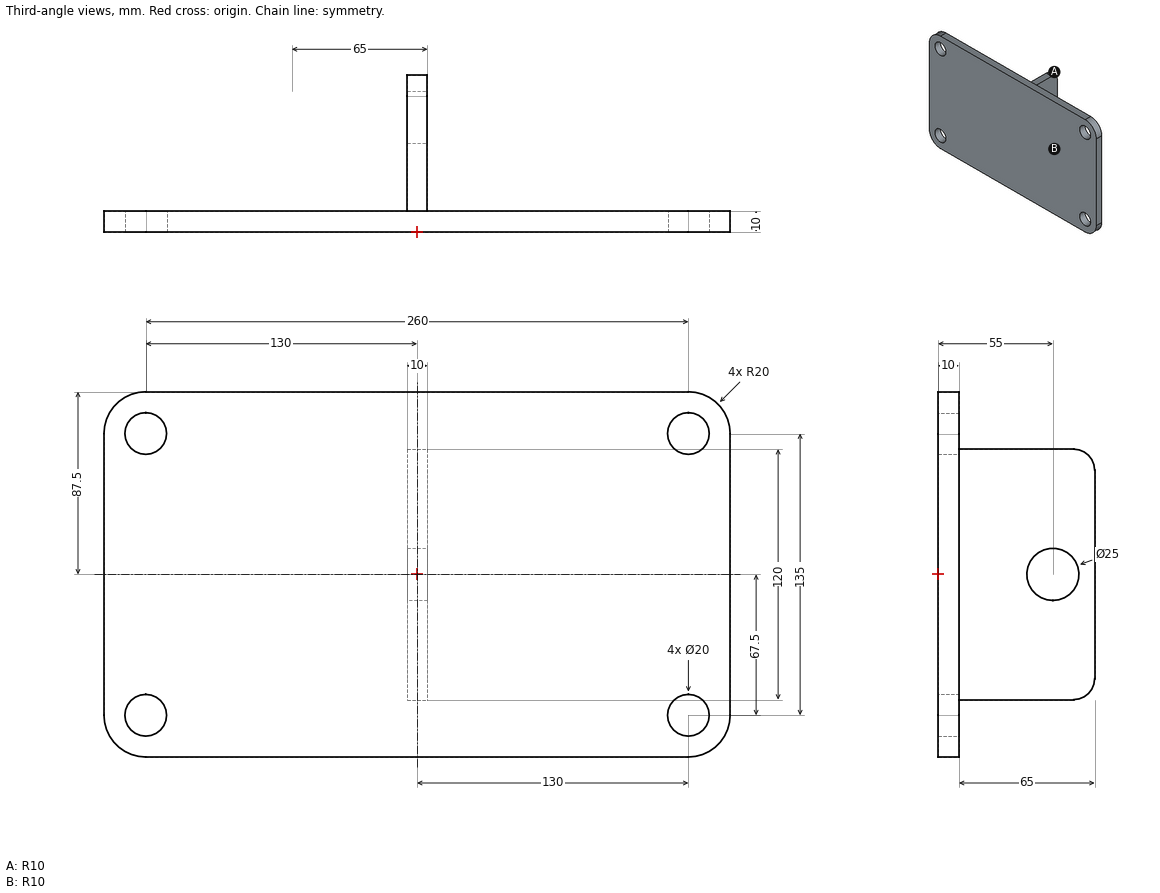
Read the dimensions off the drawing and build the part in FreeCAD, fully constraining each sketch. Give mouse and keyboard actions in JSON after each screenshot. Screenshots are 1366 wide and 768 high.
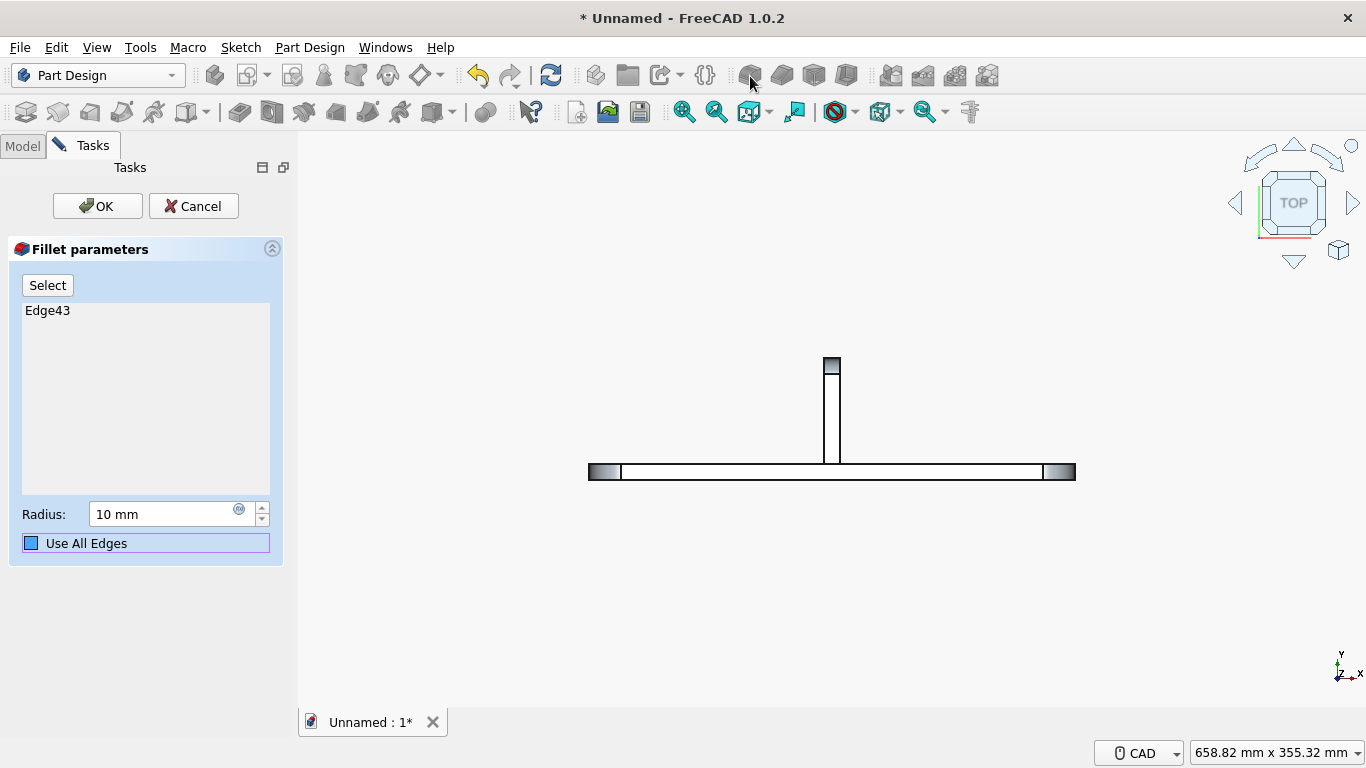
{"action": "left_click", "coordinate": [98, 206]}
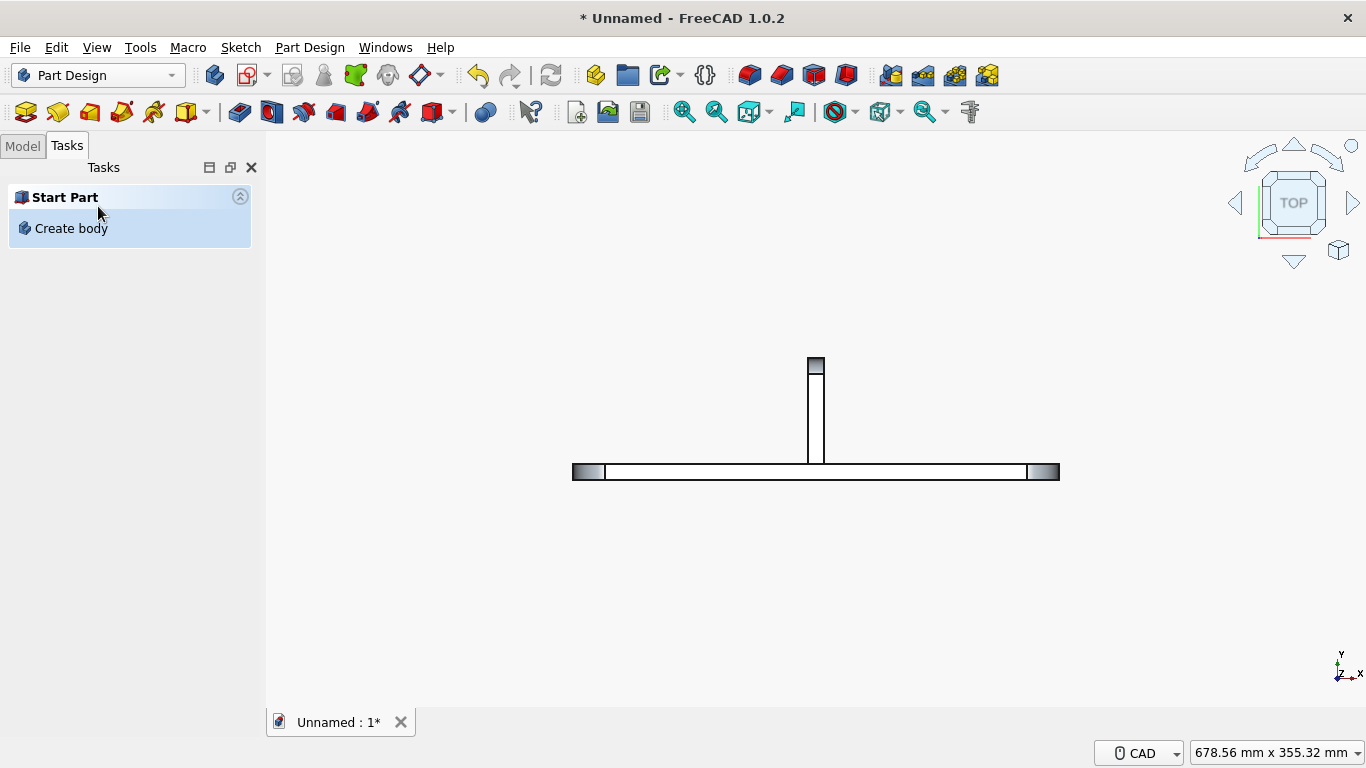
{"action": "left_click", "coordinate": [686, 112]}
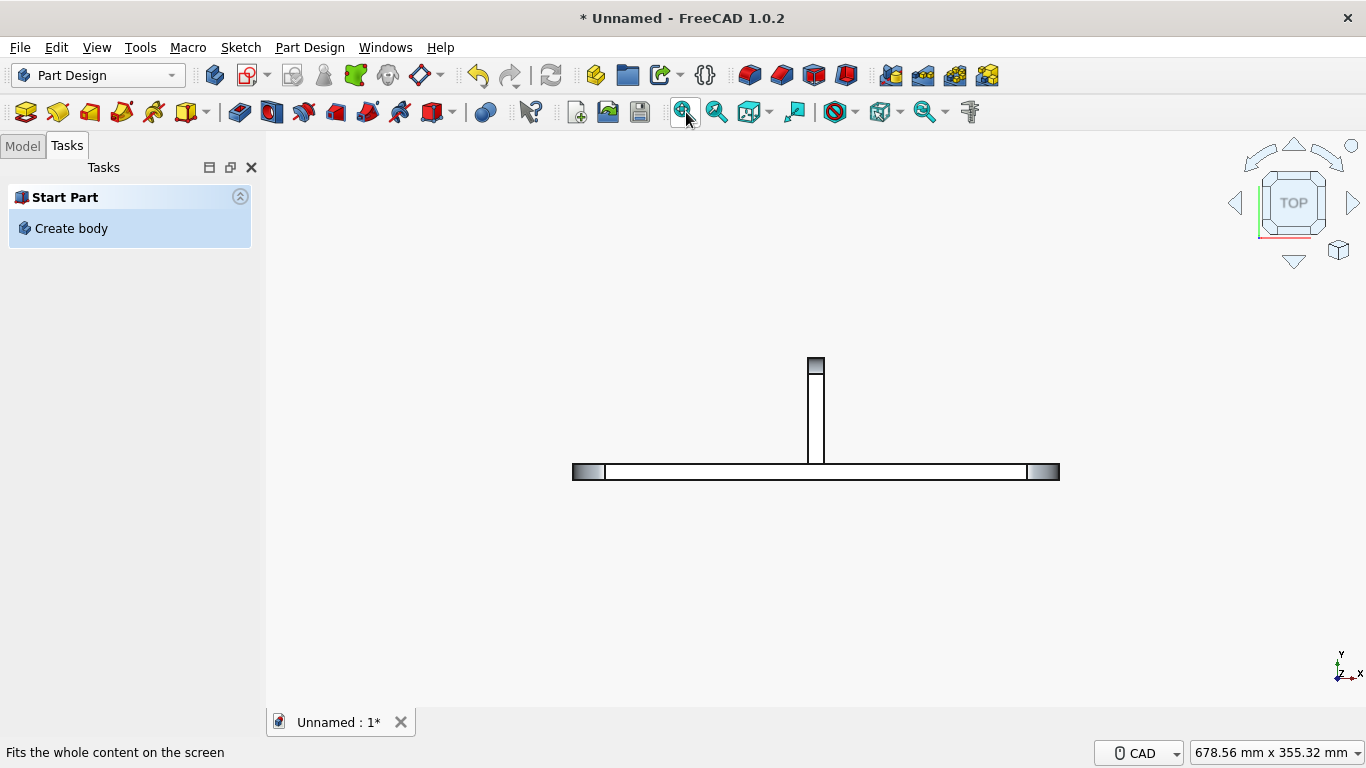
{"action": "scroll", "coordinate": [816, 357], "scroll_direction": "up", "scroll_amount": 5}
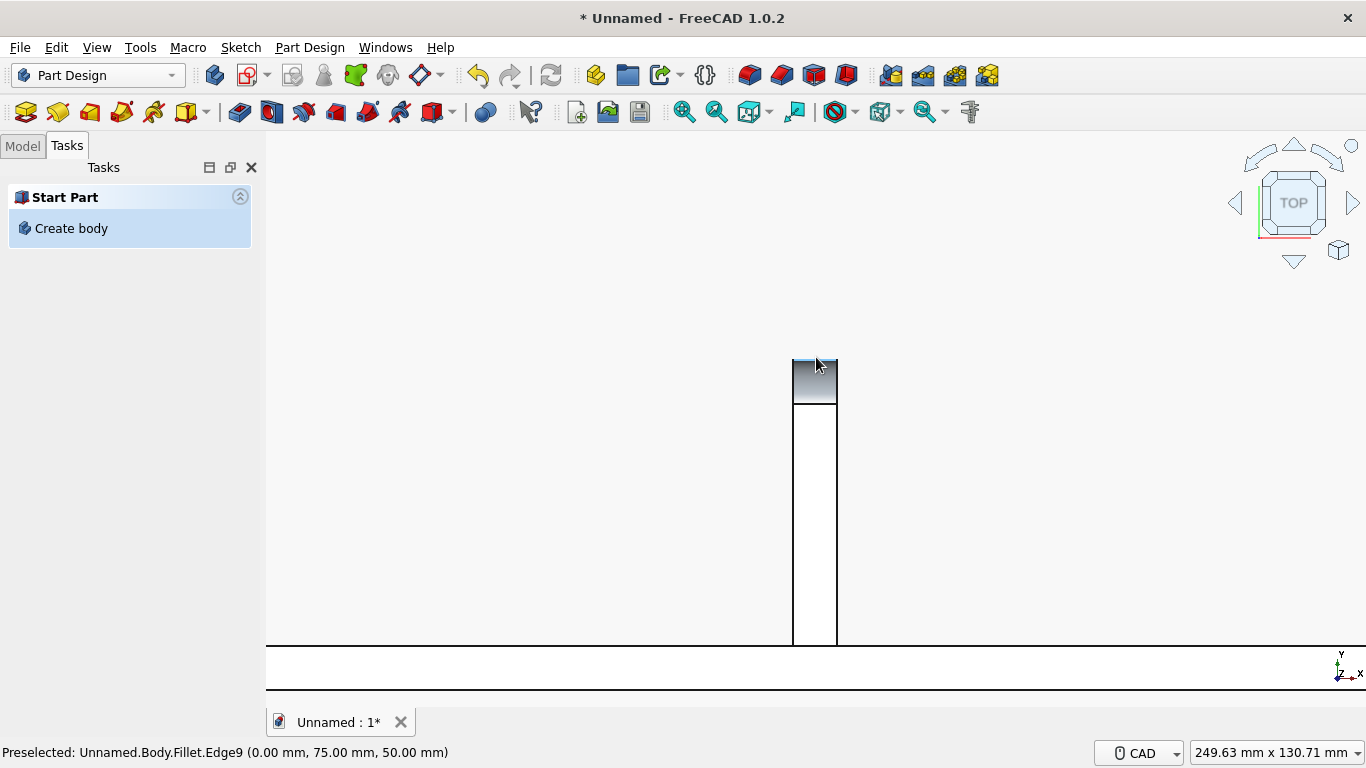
{"action": "left_click", "coordinate": [686, 112]}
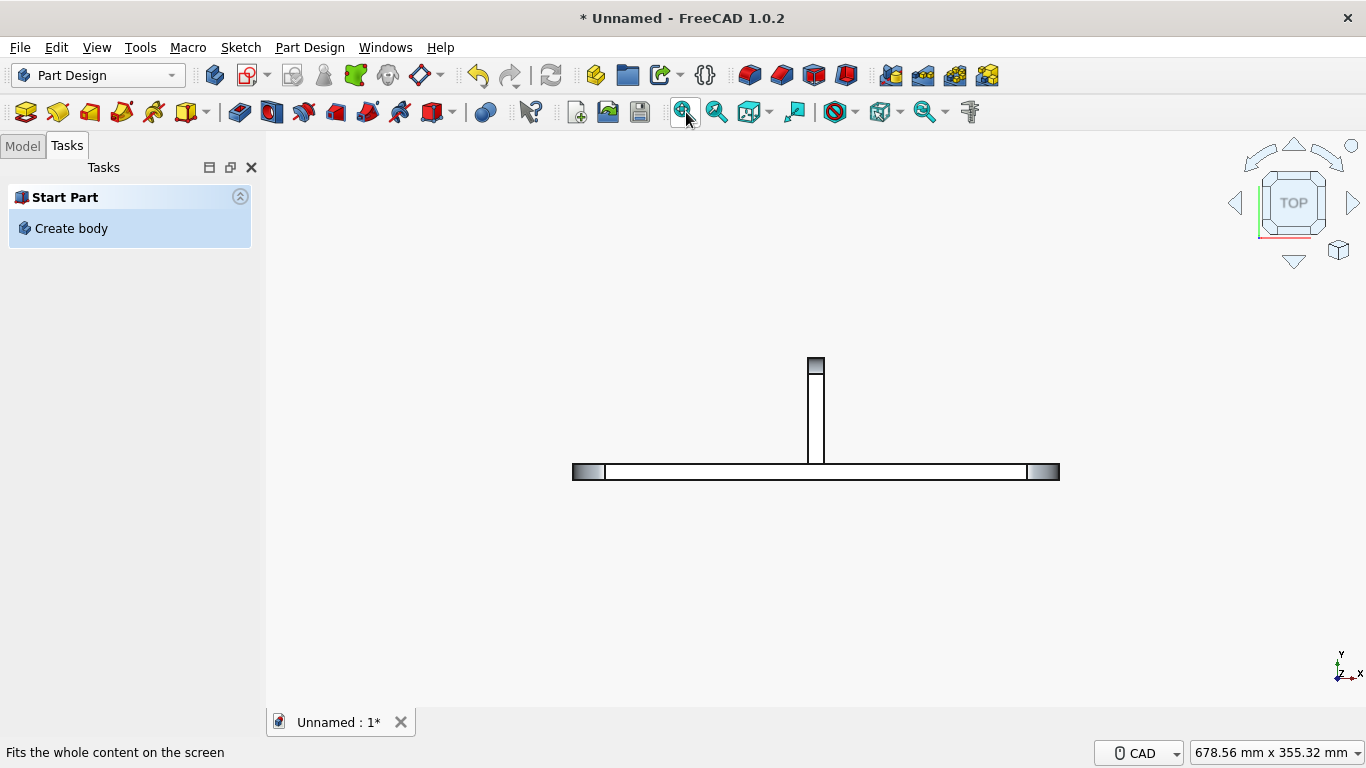
{"action": "key", "text": "0"}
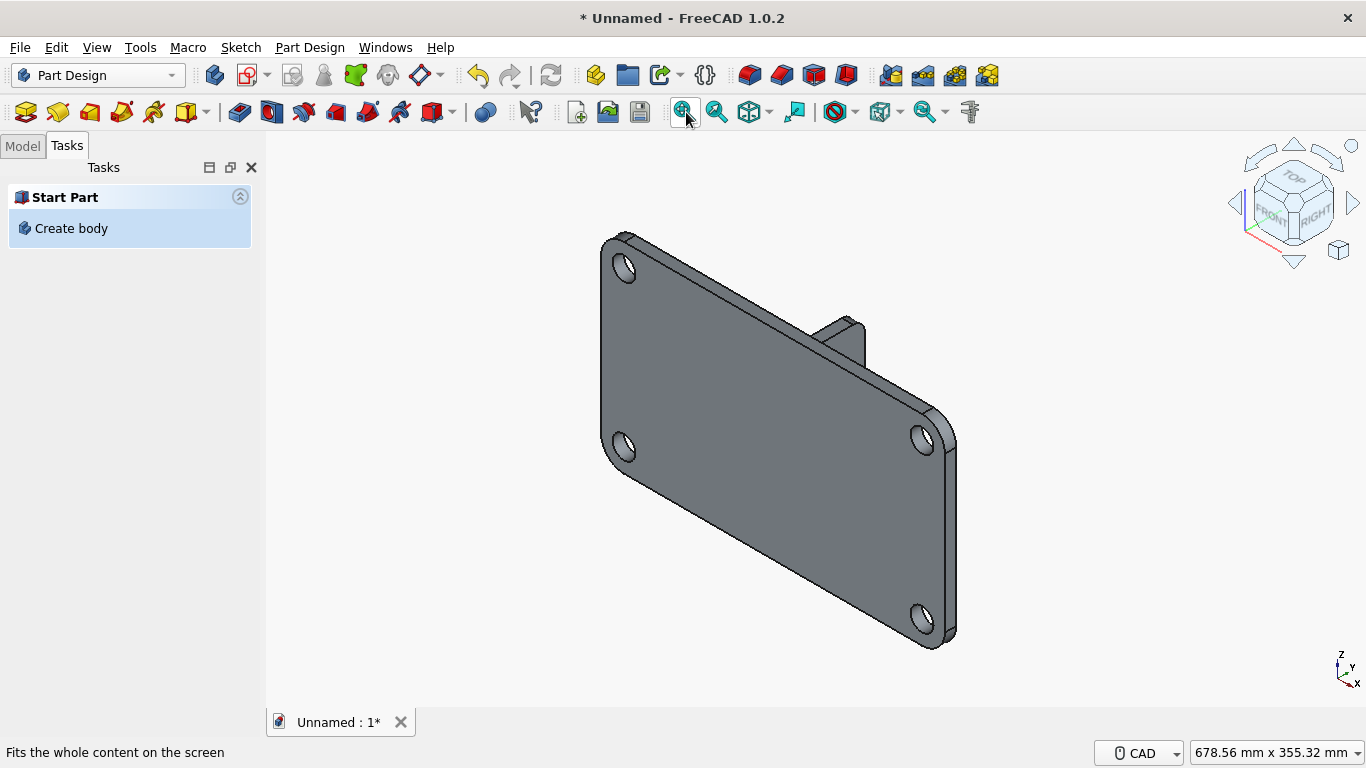
{"action": "scroll", "coordinate": [859, 473], "scroll_direction": "up", "scroll_amount": 5}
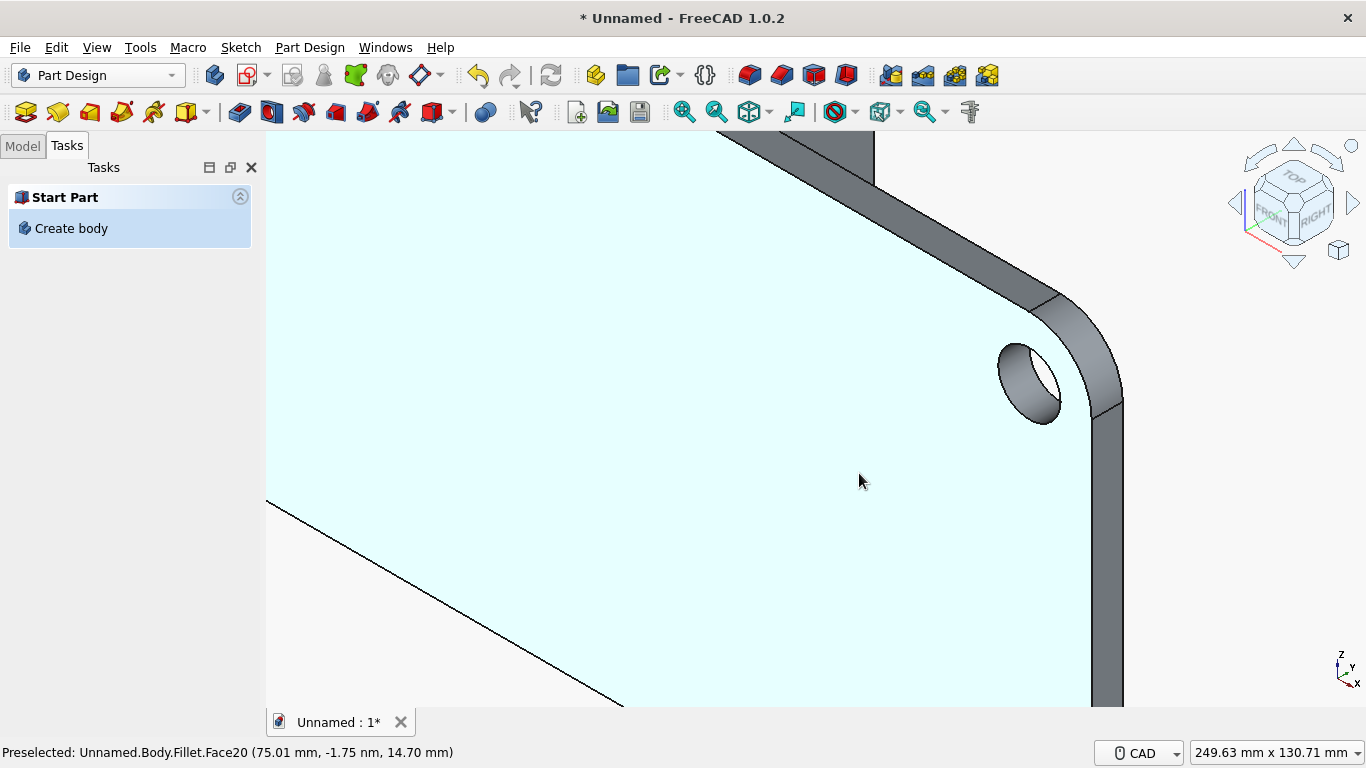
{"action": "left_click", "coordinate": [686, 112]}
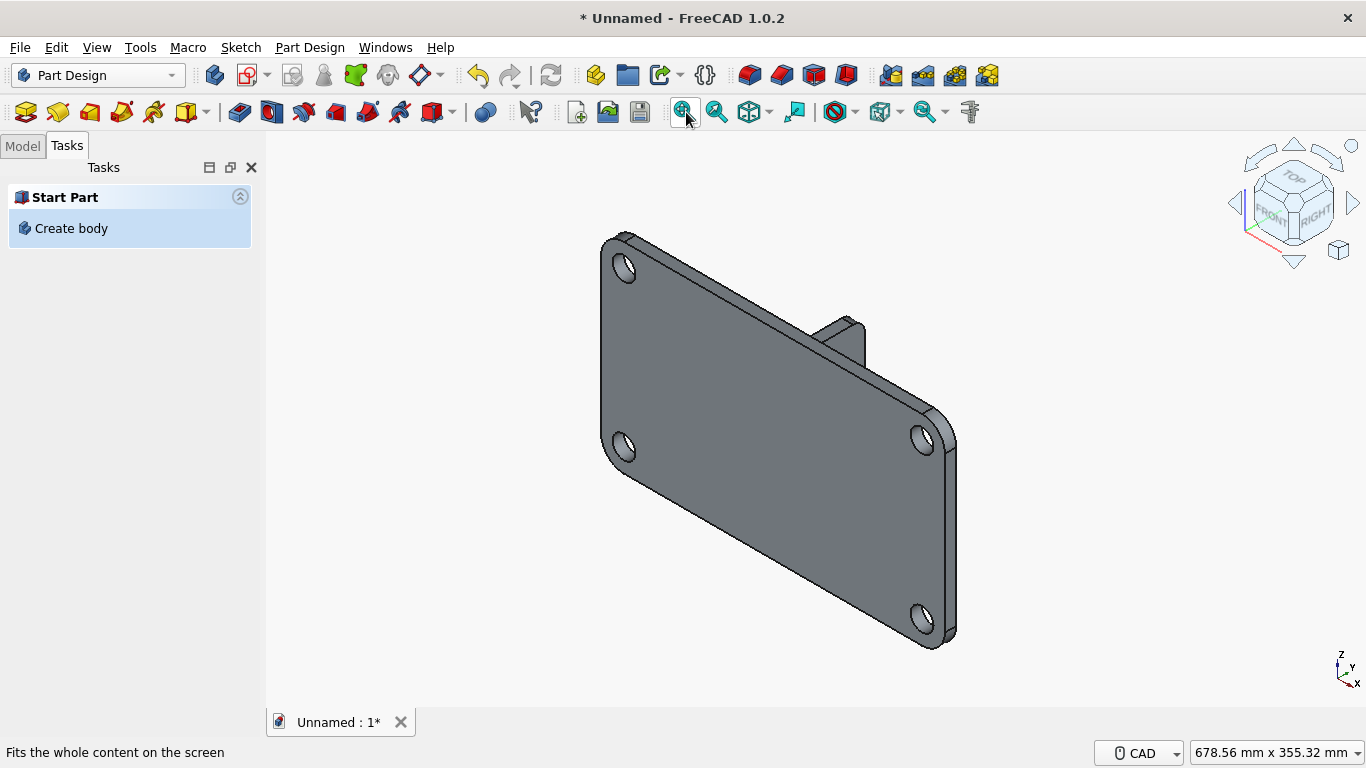
{"action": "key", "text": "2"}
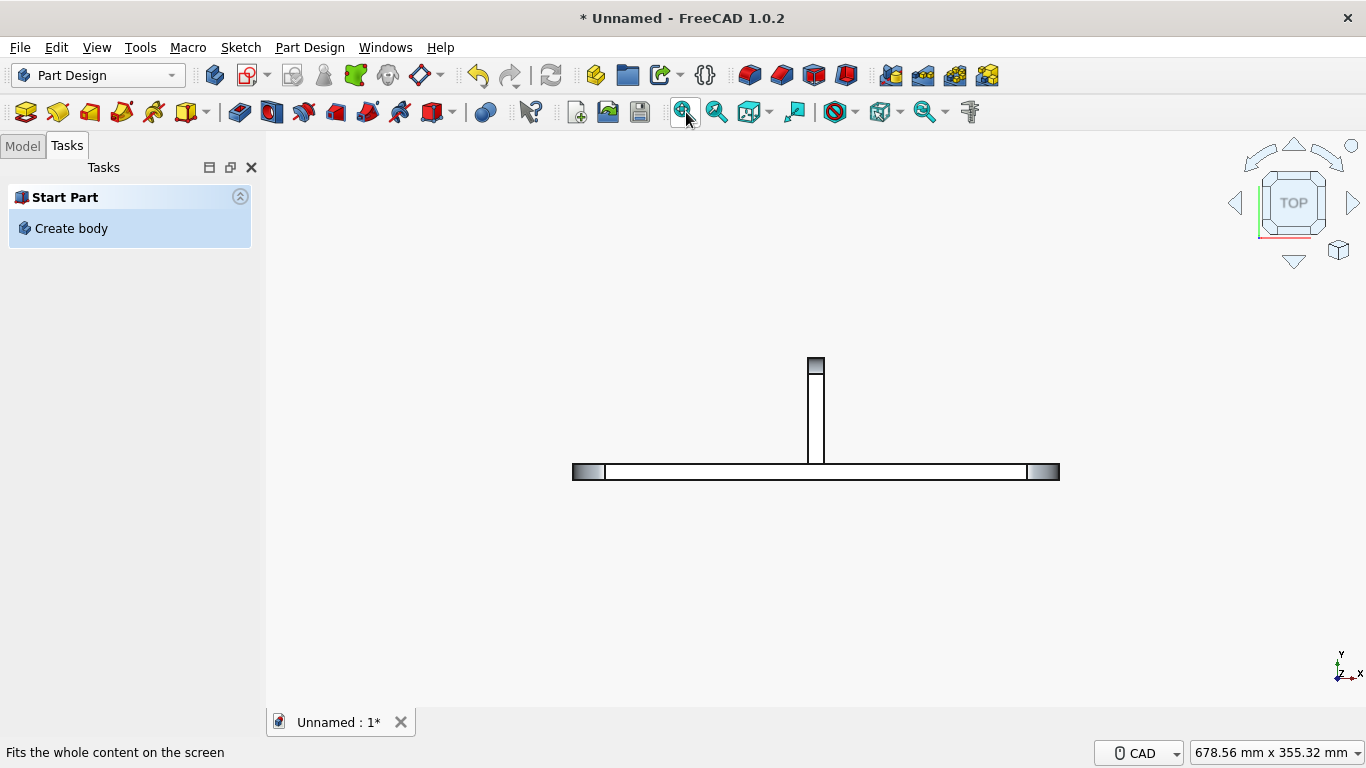
{"action": "left_click", "coordinate": [686, 112]}